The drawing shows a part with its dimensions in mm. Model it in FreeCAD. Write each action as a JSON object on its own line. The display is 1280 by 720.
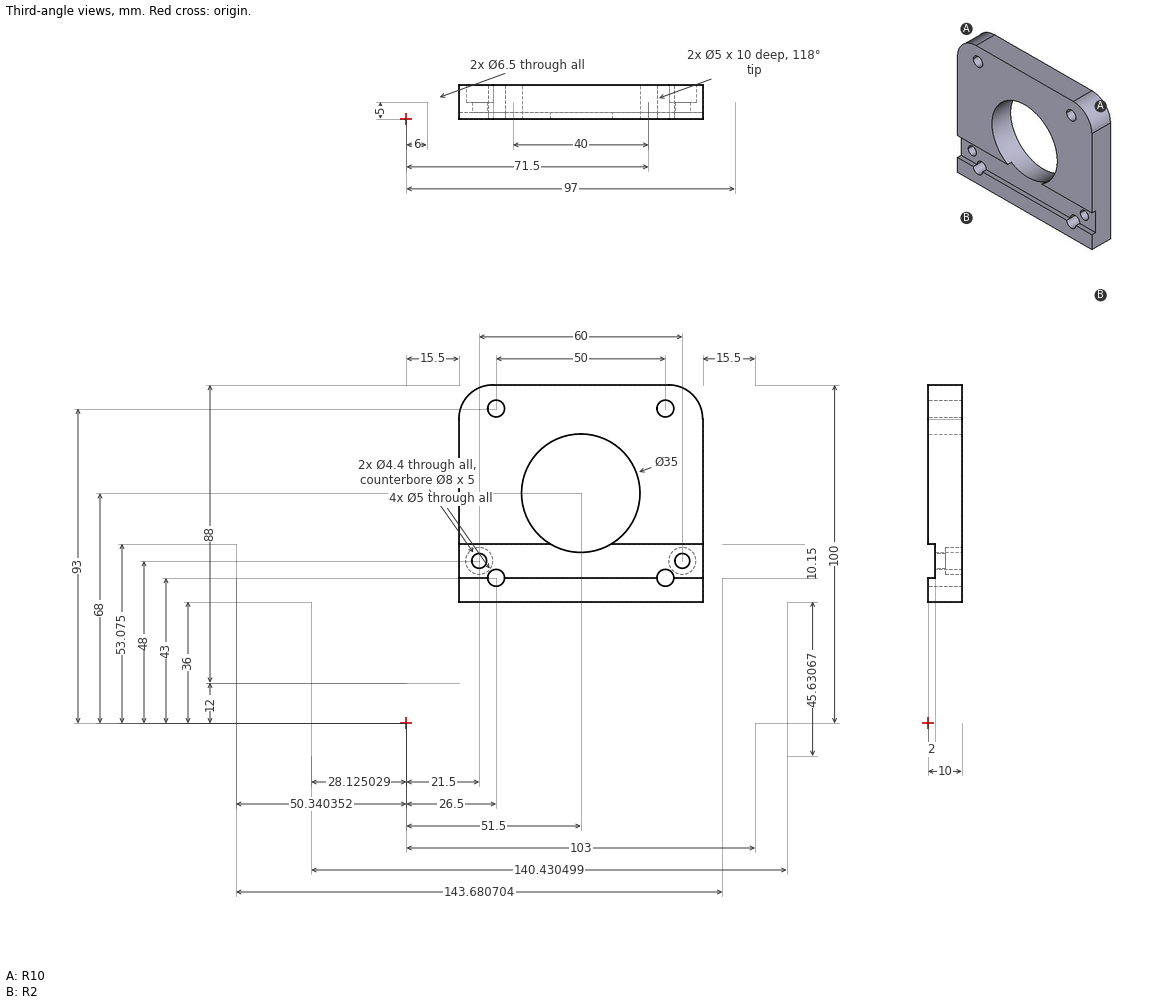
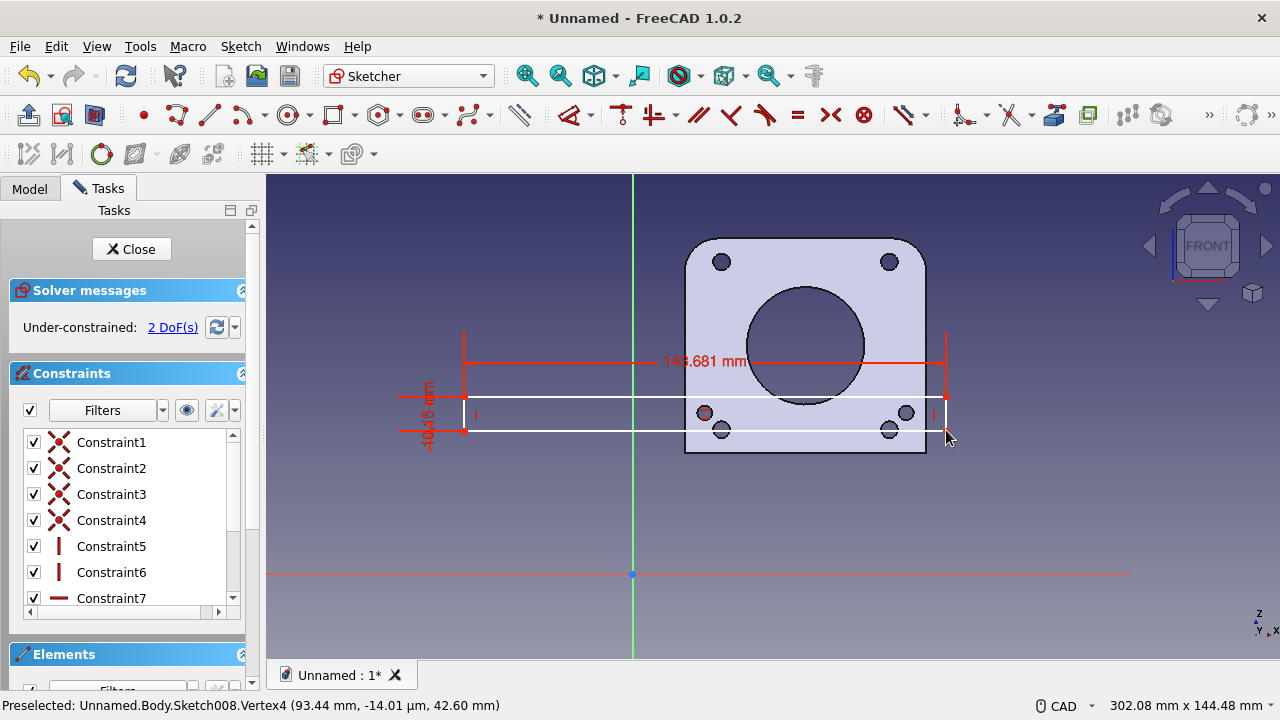
{"action": "key", "text": "d"}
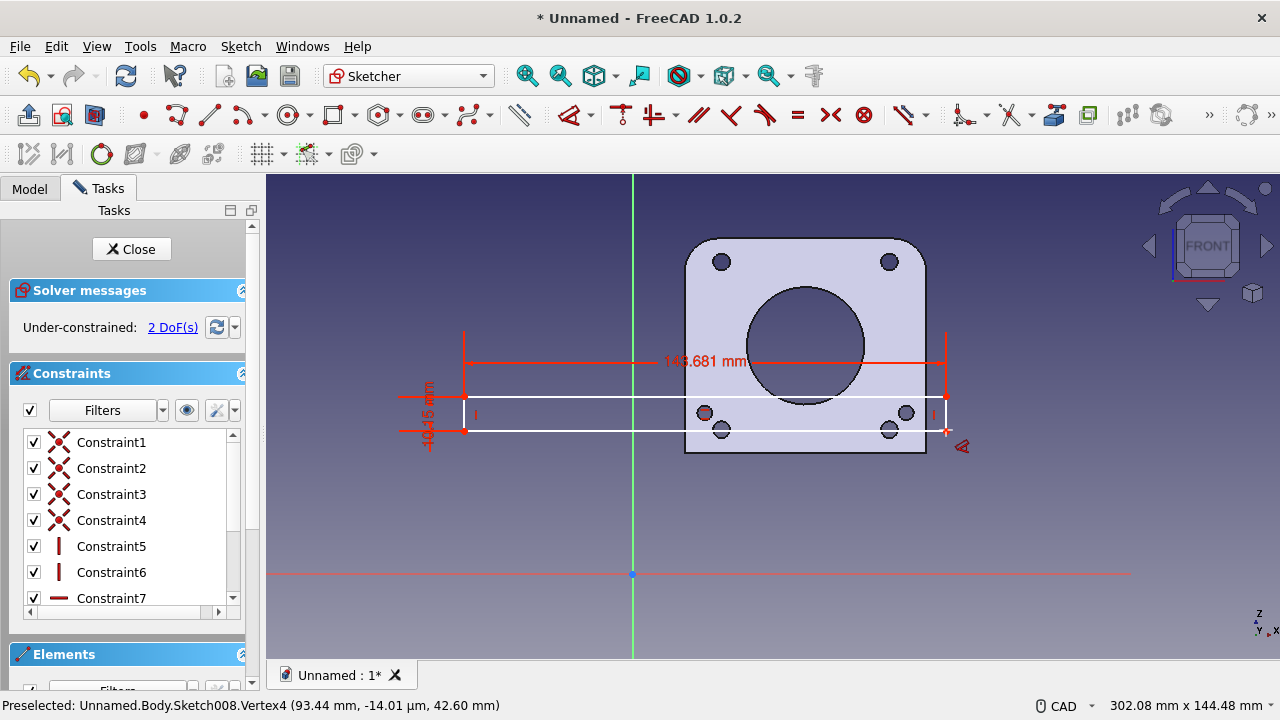
{"action": "left_click", "coordinate": [464, 397]}
{"action": "left_click", "coordinate": [430, 486]}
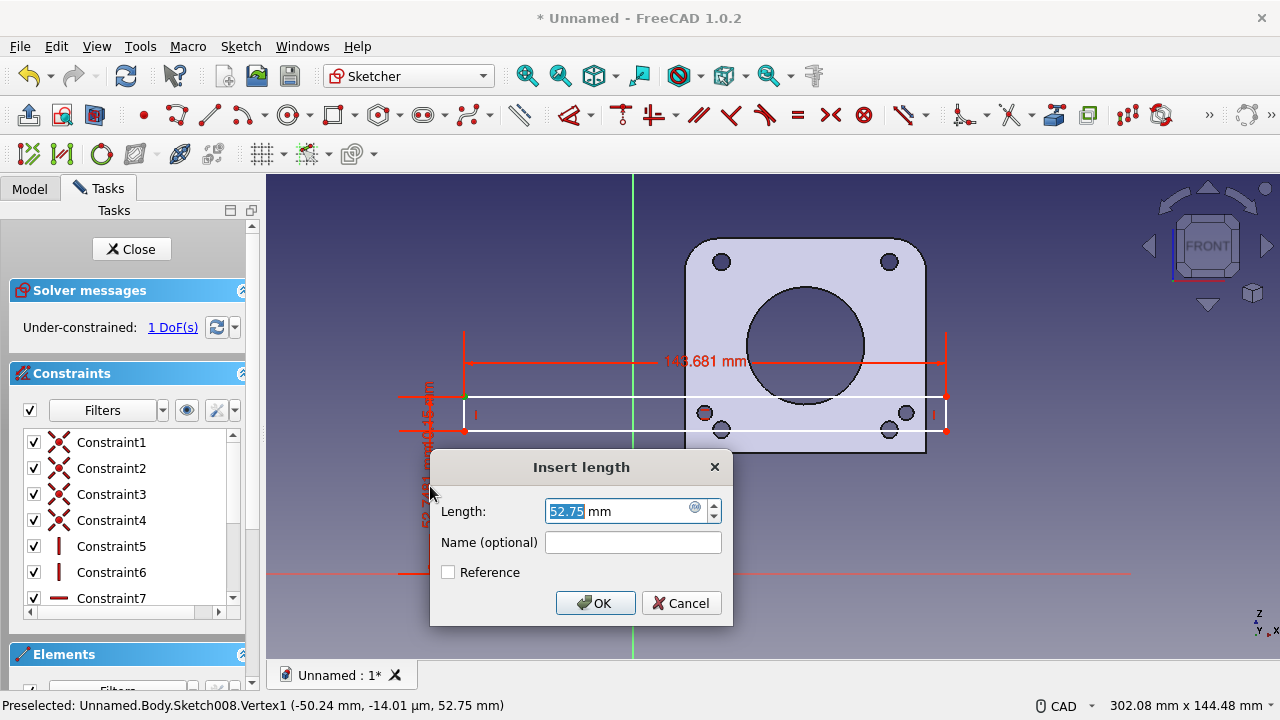
{"action": "type", "text": "53.075"}
{"action": "key", "text": "Return"}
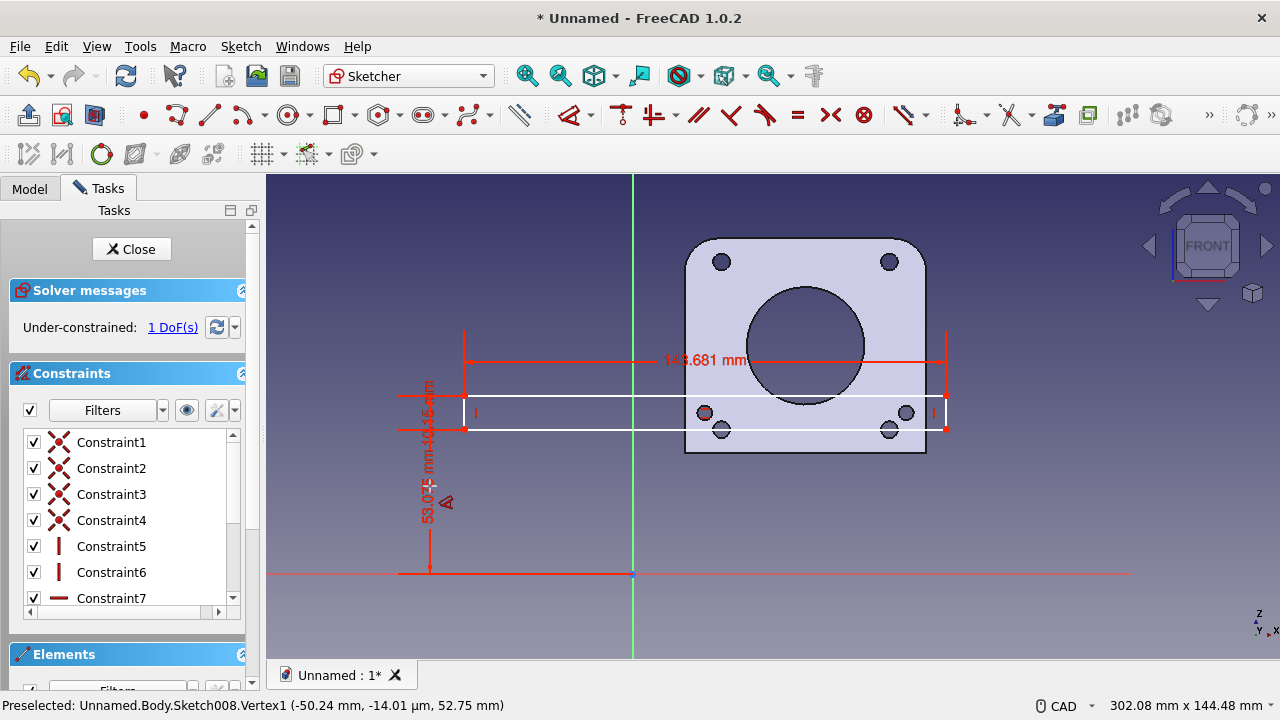
{"action": "left_click", "coordinate": [464, 396]}
{"action": "left_click", "coordinate": [548, 608]}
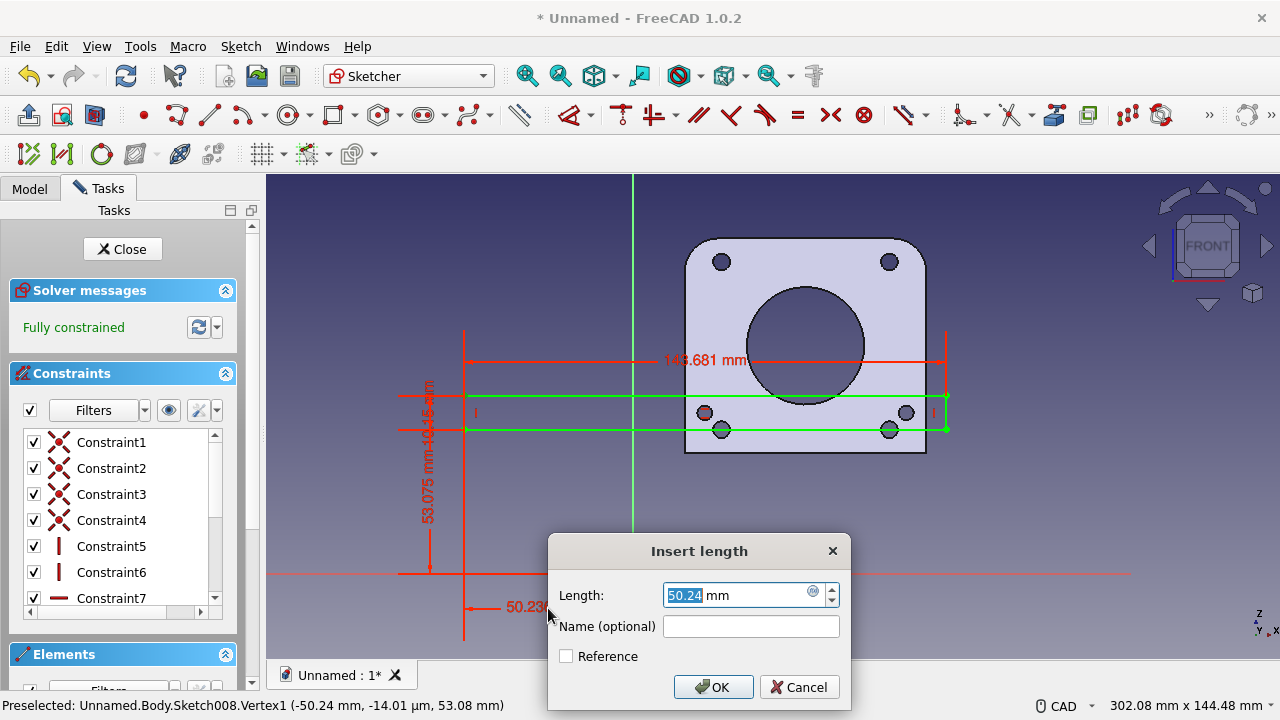
{"action": "type", "text": "50.340352"}
{"action": "key", "text": "Return"}
{"action": "key", "text": "Escape"}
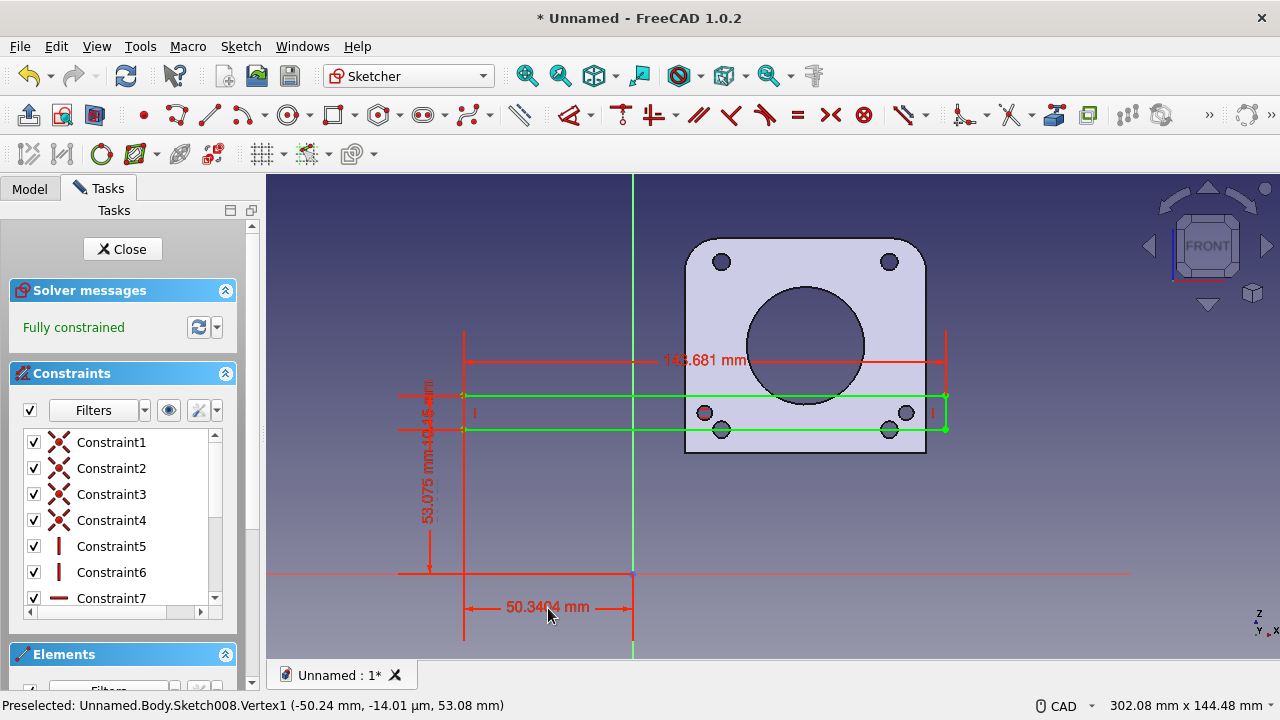
{"action": "left_click", "coordinate": [123, 249]}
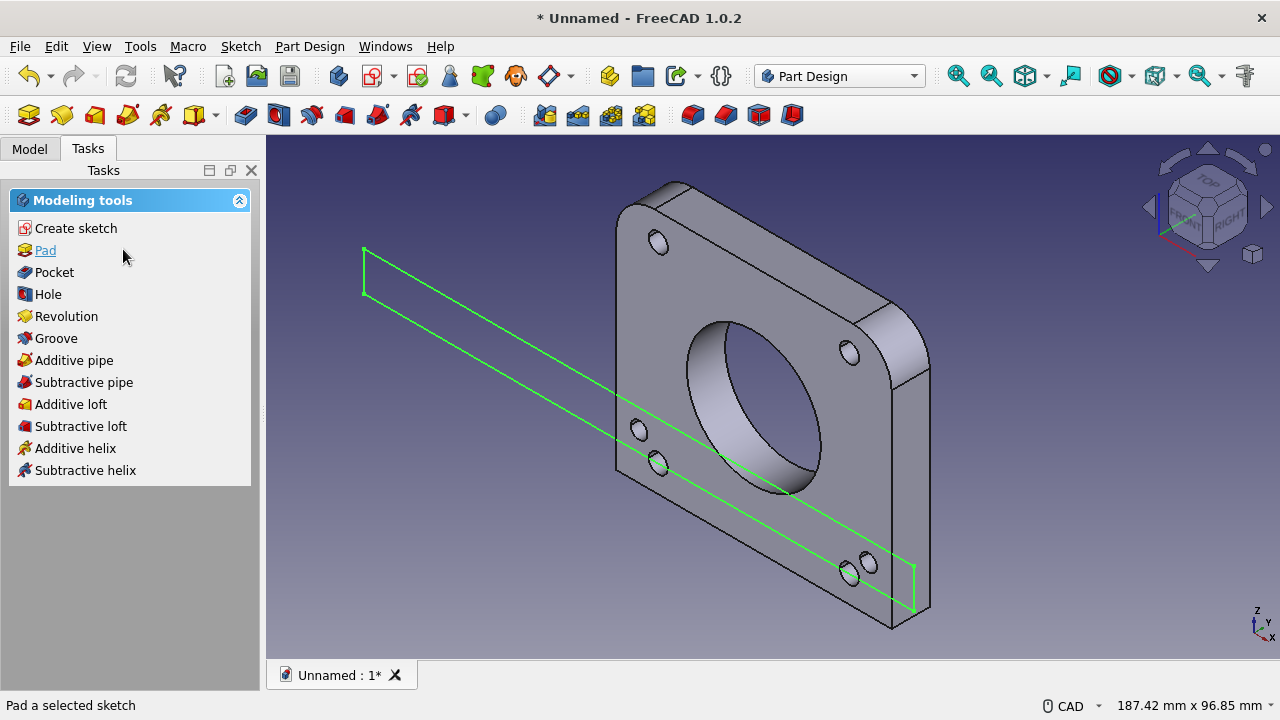
{"action": "left_click", "coordinate": [246, 116]}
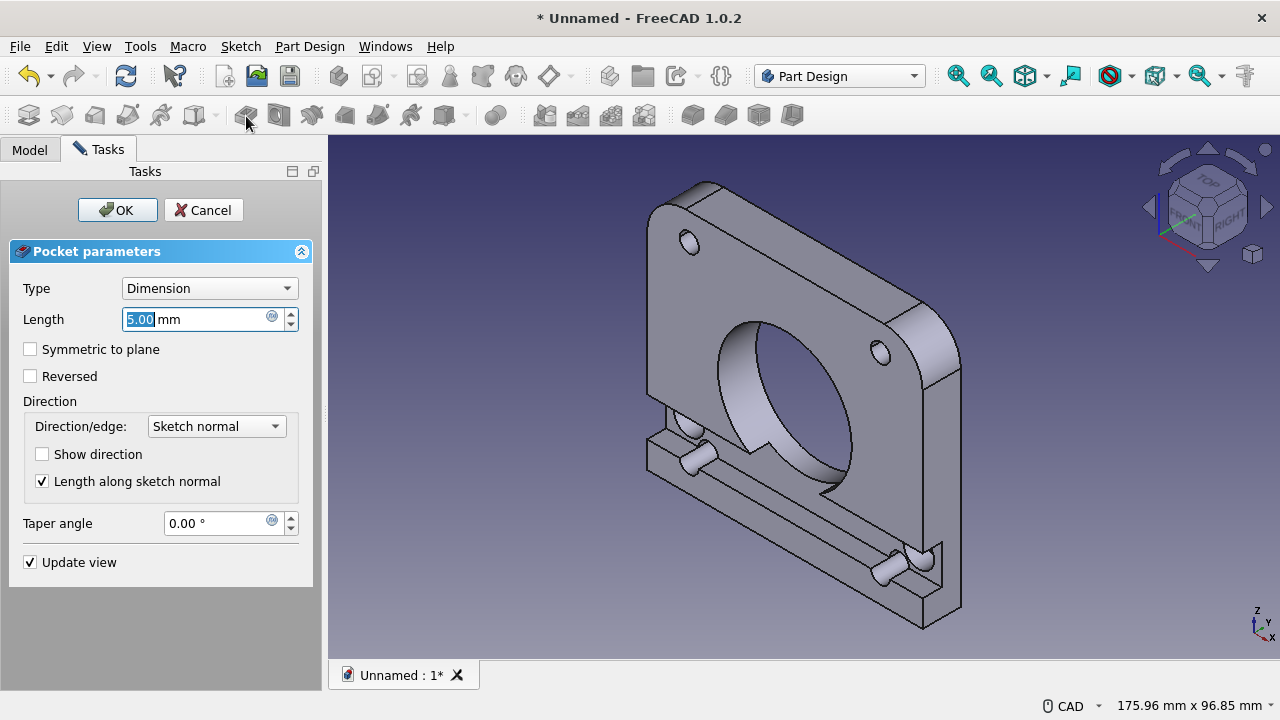
{"action": "type", "text": "2"}
{"action": "key", "text": "Tab"}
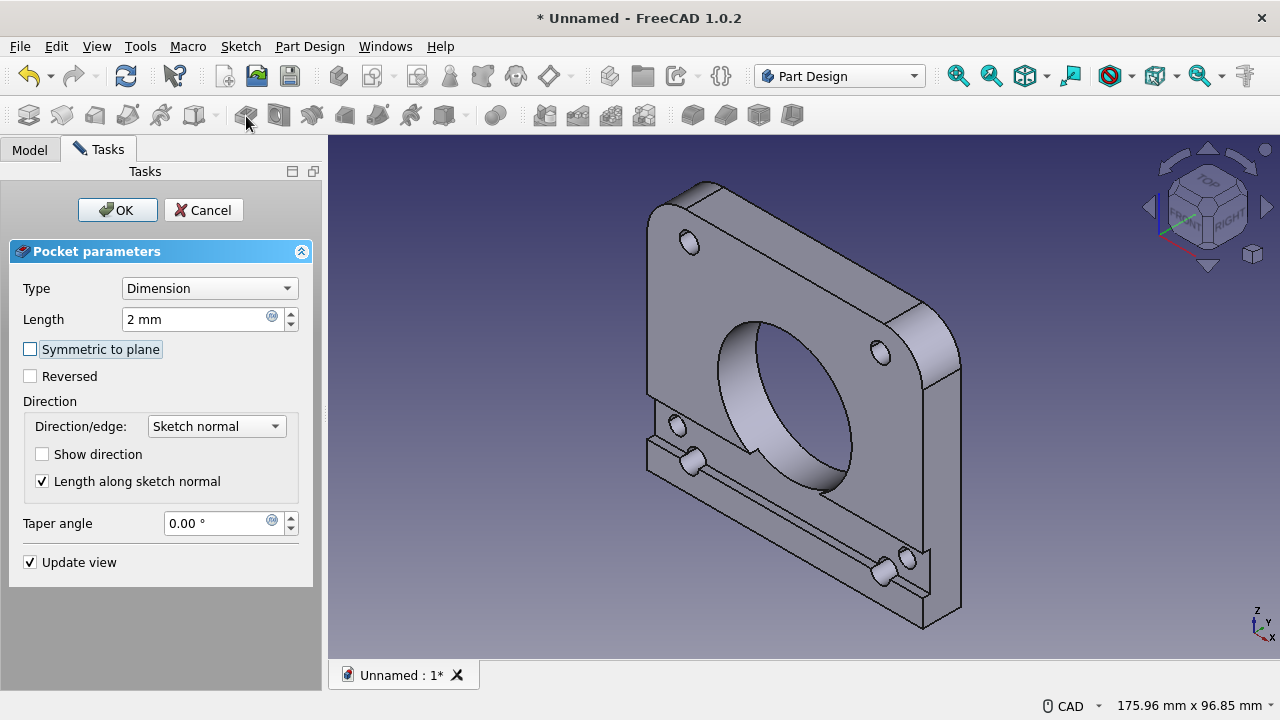
{"action": "left_click", "coordinate": [118, 210]}